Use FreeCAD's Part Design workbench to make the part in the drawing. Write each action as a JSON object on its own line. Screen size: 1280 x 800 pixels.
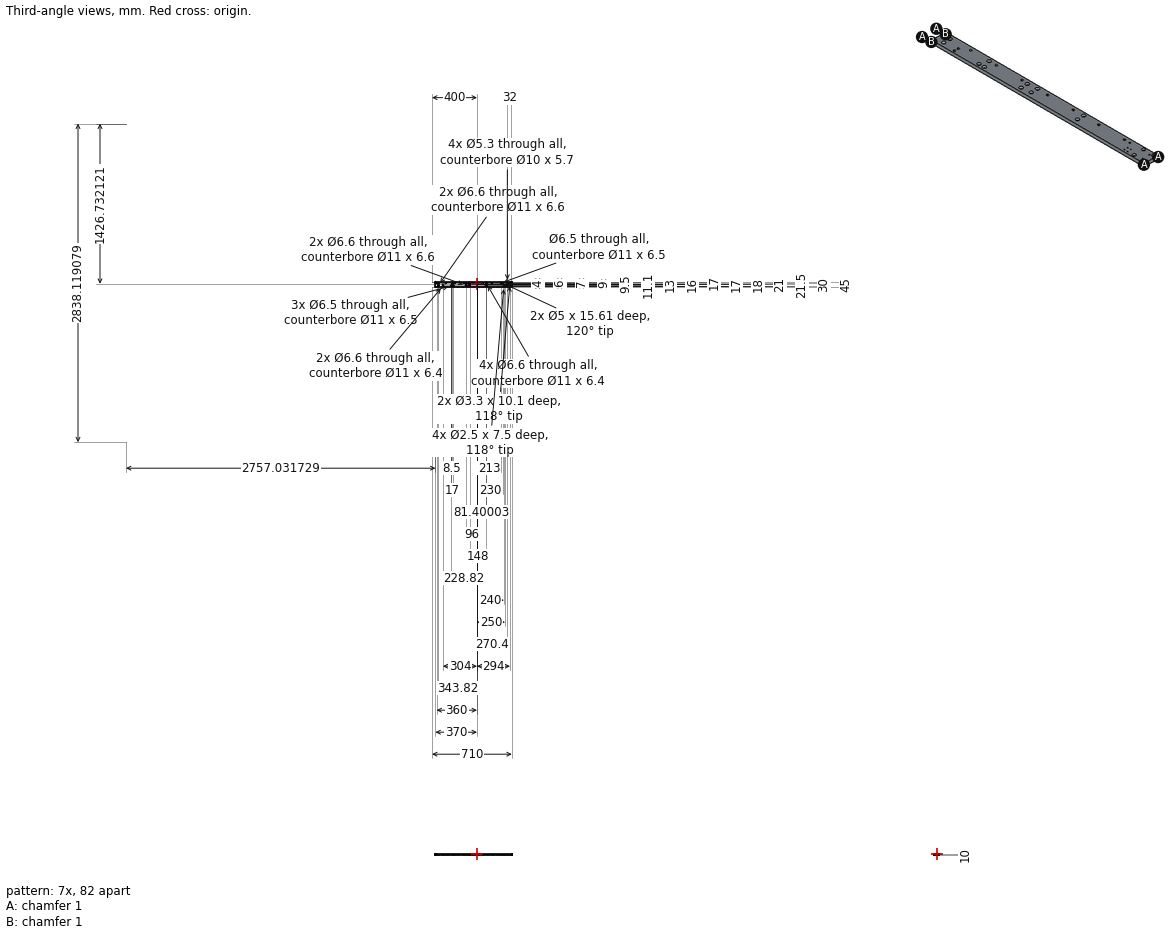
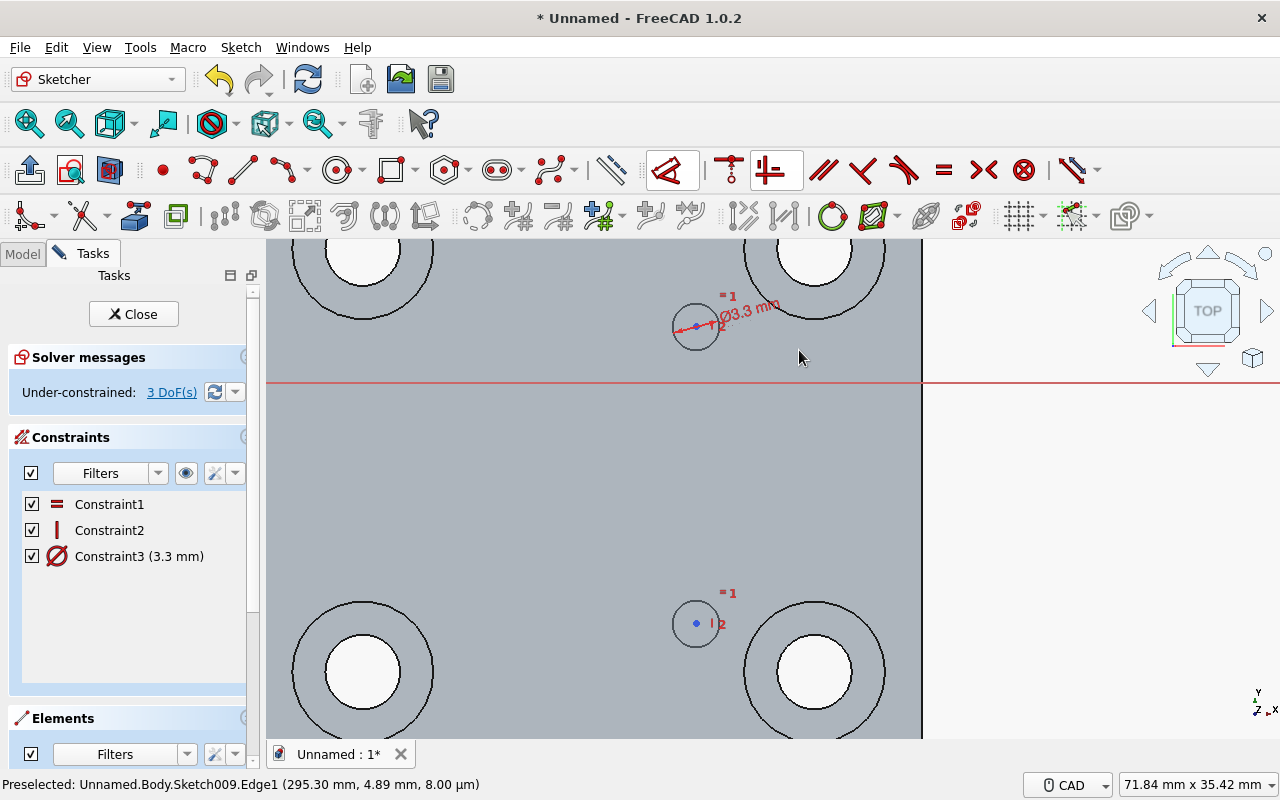
{"action": "left_click", "coordinate": [696, 327]}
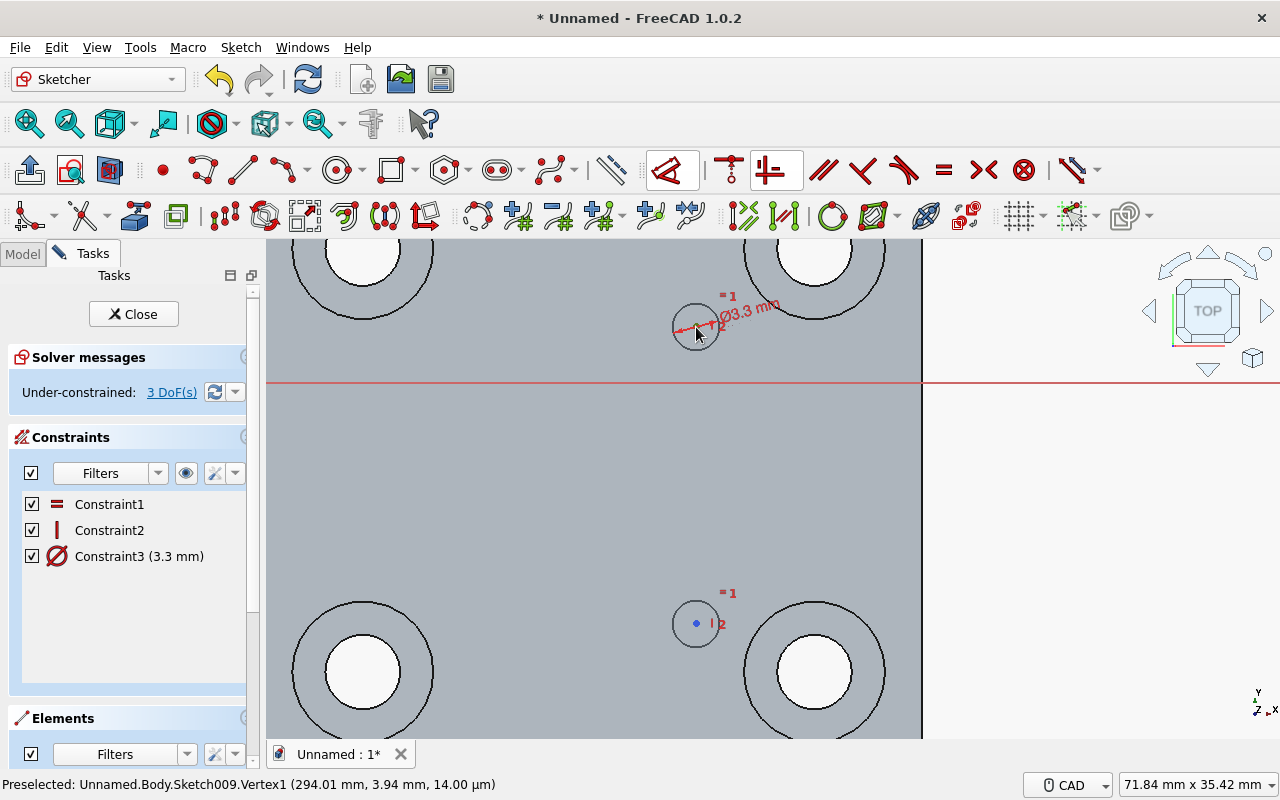
{"action": "left_click", "coordinate": [694, 170]}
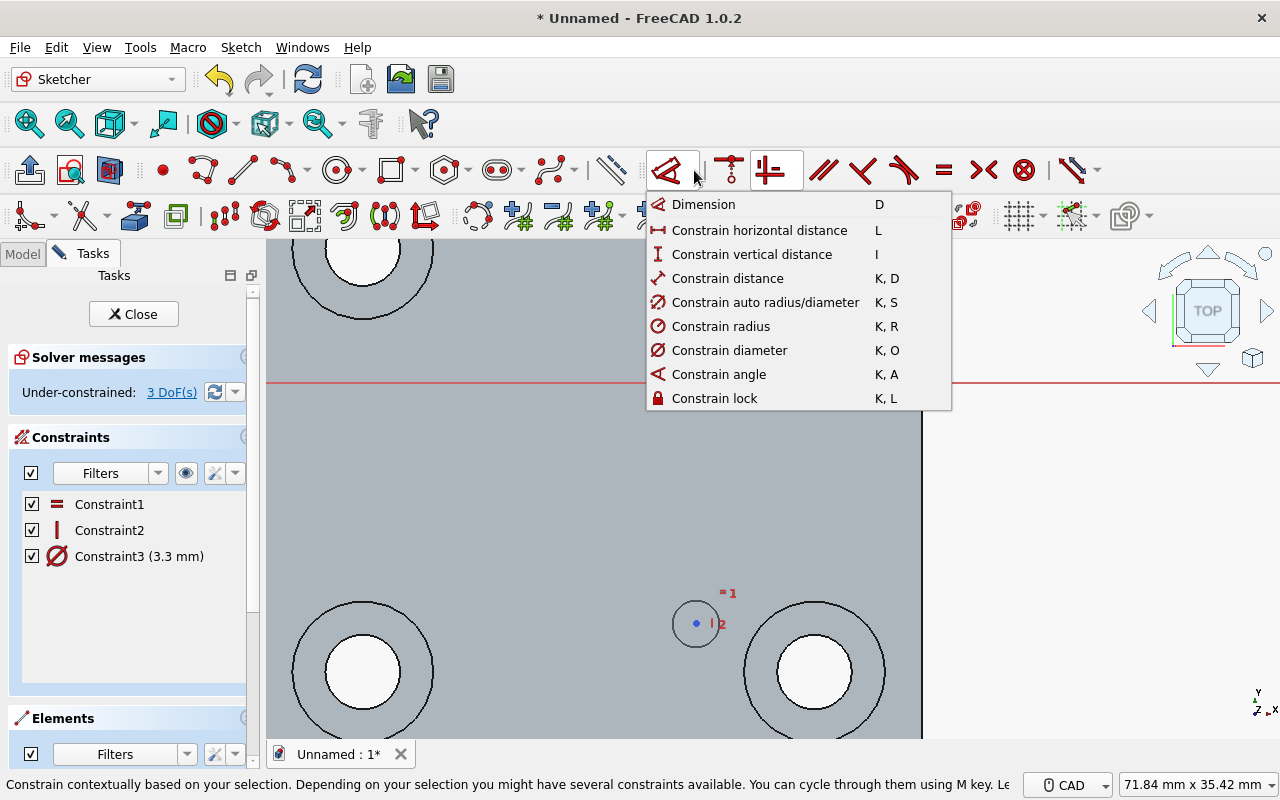
{"action": "left_click", "coordinate": [799, 254]}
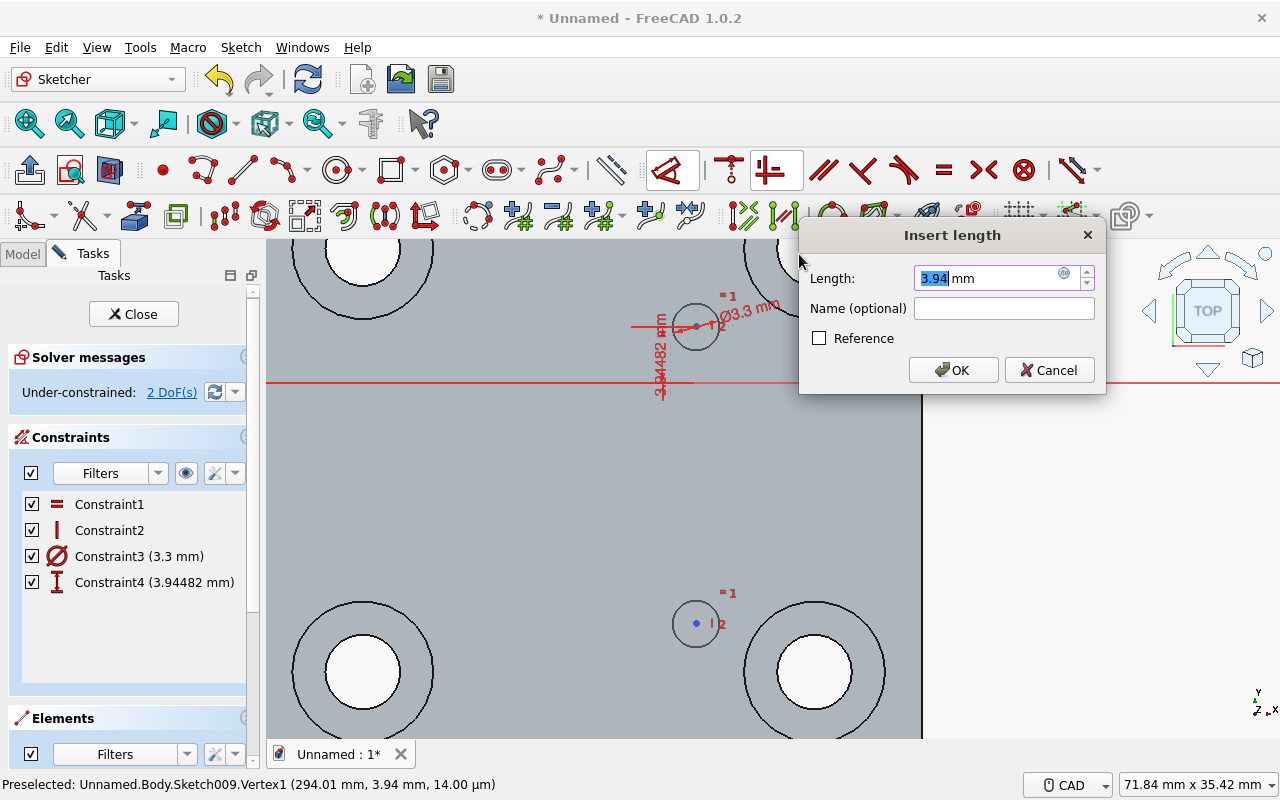
{"action": "type", "text": "4"}
{"action": "key", "text": "Return"}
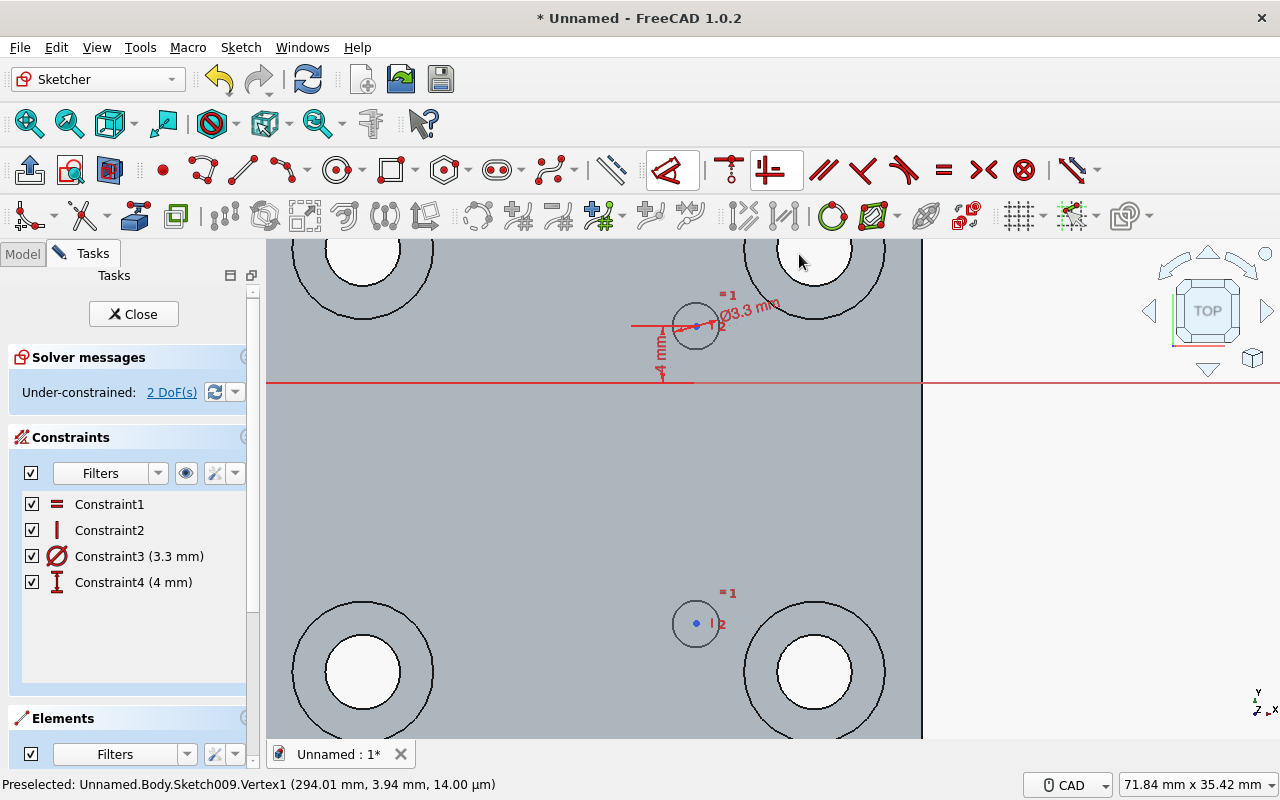
{"action": "left_click", "coordinate": [696, 624]}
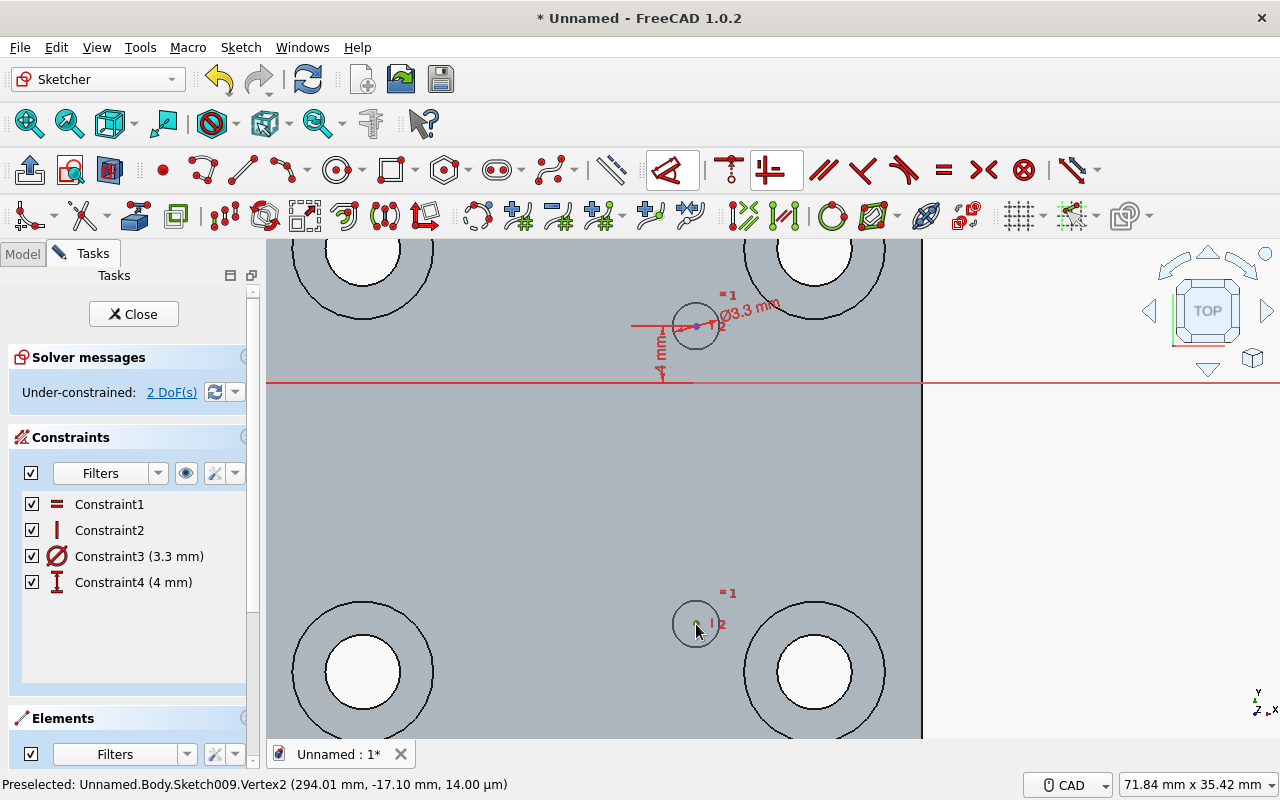
{"action": "left_click", "coordinate": [694, 170]}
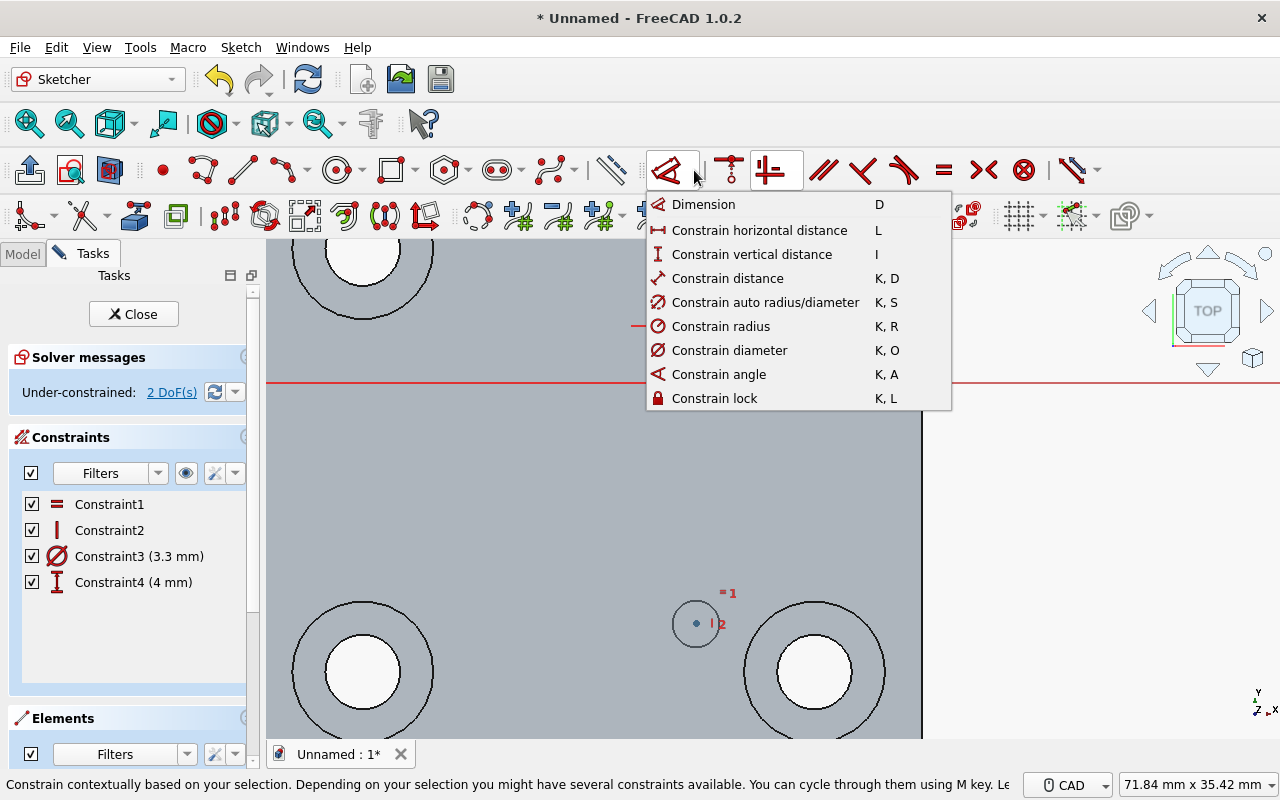
{"action": "left_click", "coordinate": [799, 254]}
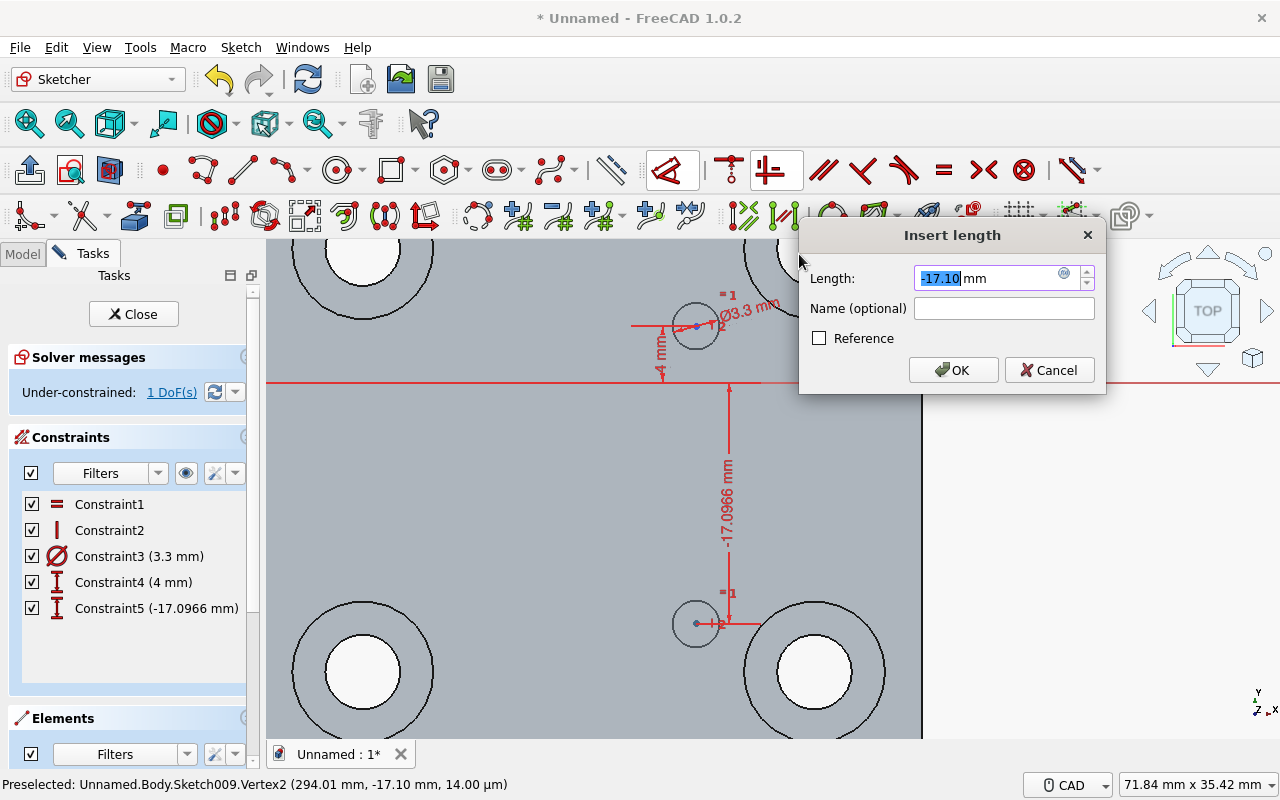
{"action": "type", "text": "-17"}
{"action": "key", "text": "Return"}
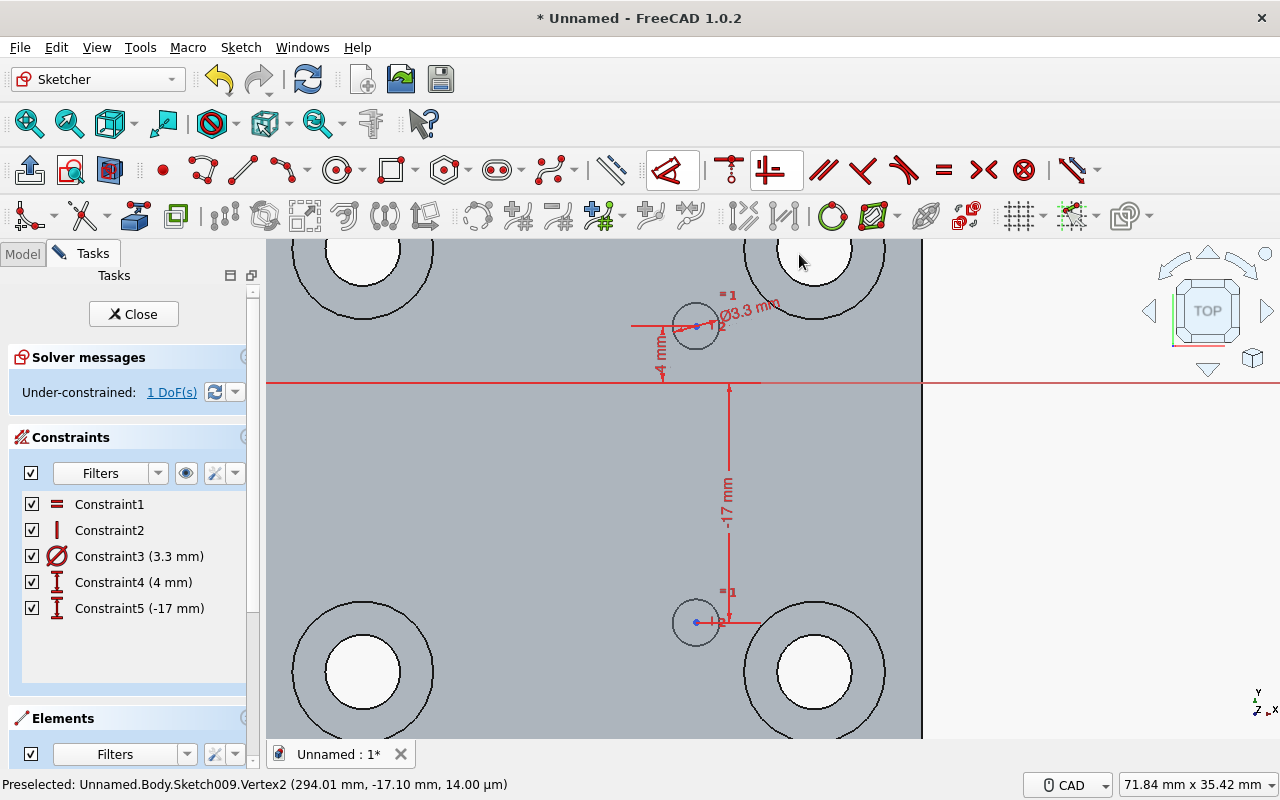
{"action": "left_click", "coordinate": [696, 326]}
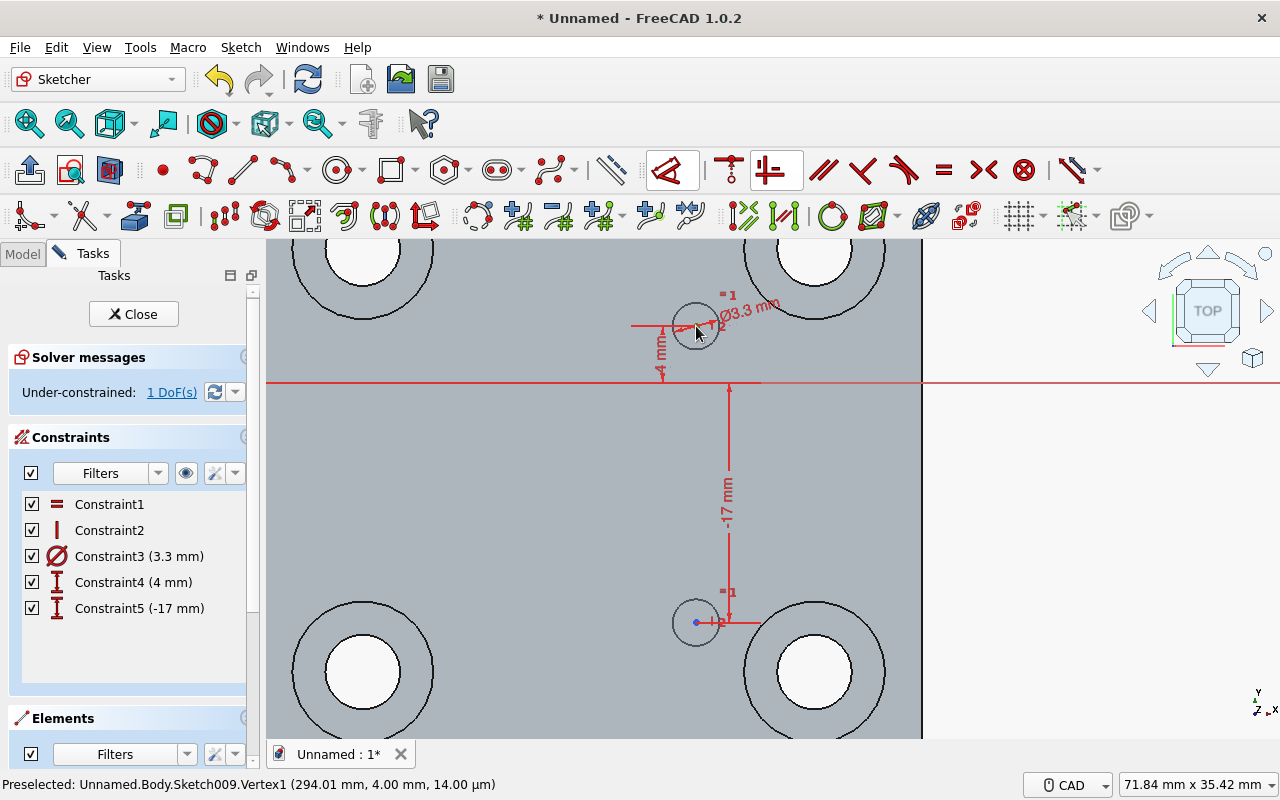
{"action": "key", "text": "l"}